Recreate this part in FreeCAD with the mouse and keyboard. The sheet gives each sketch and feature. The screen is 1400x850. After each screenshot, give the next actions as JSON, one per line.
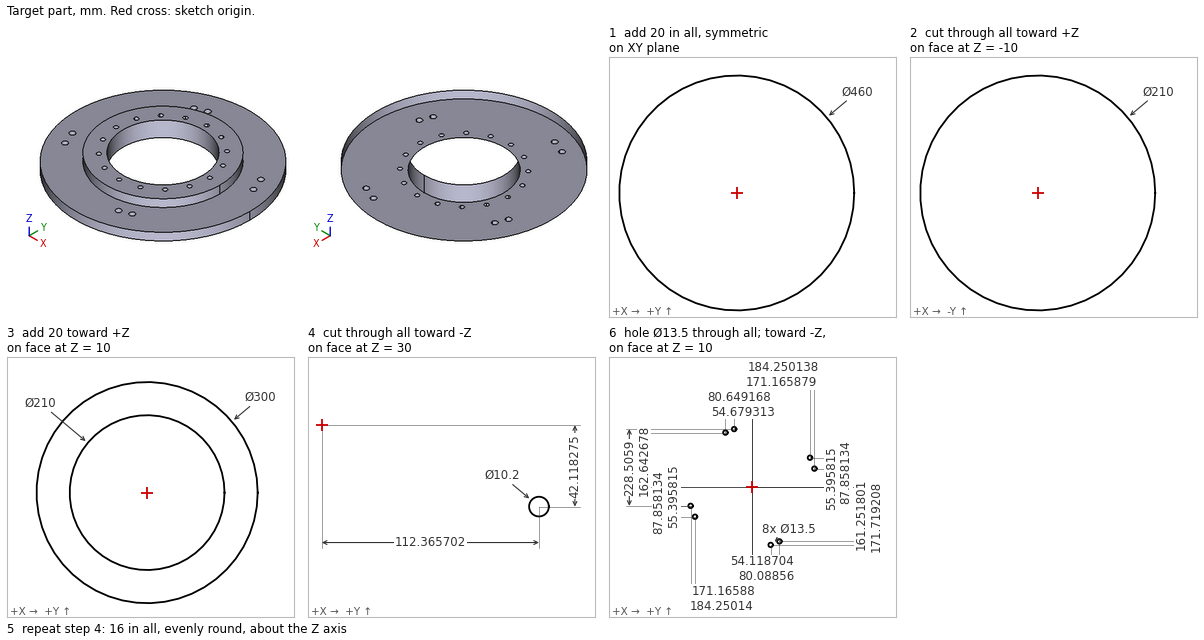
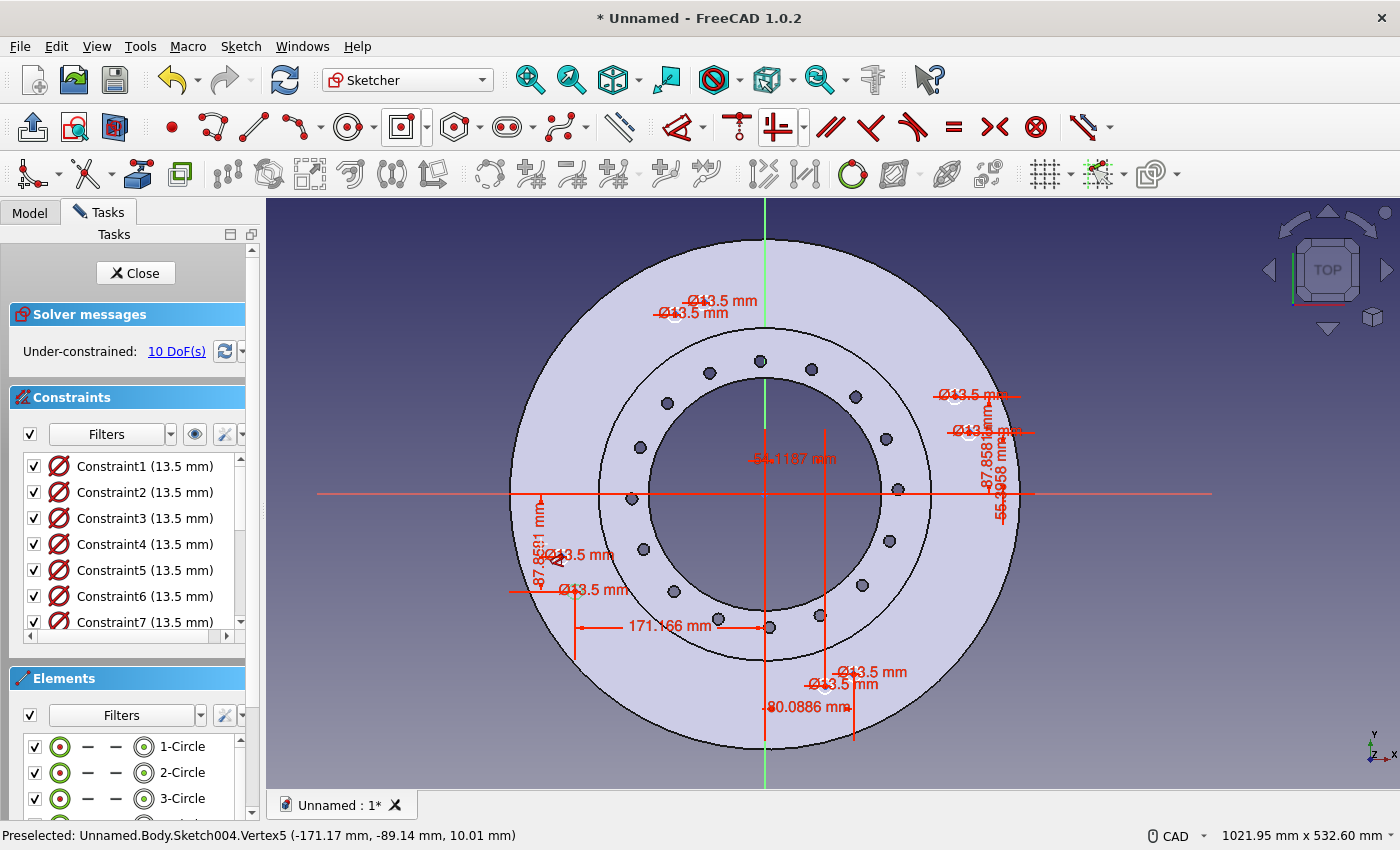
{"action": "left_click", "coordinate": [561, 557]}
{"action": "left_click", "coordinate": [663, 591]}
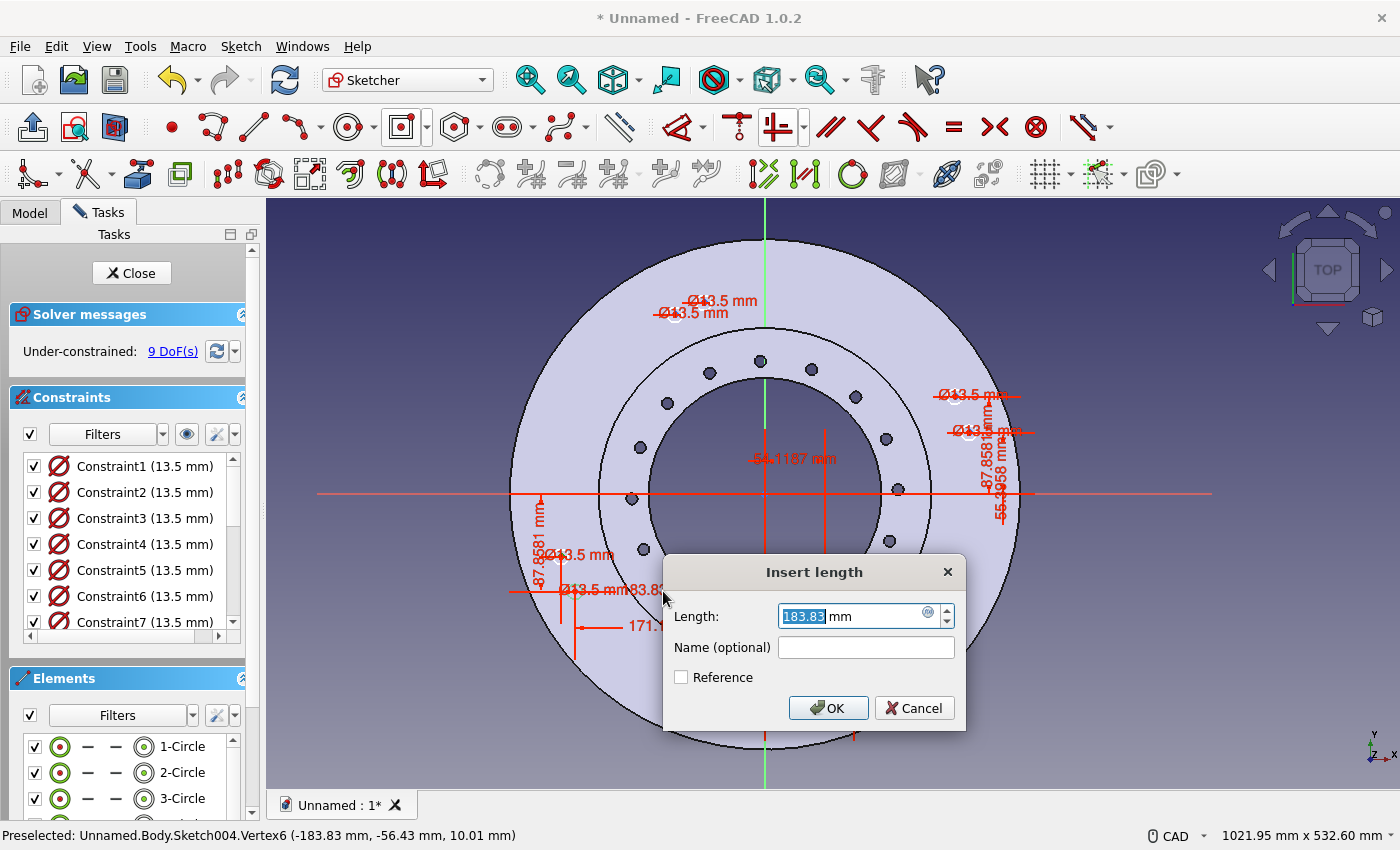
{"action": "type", "text": "184.25014"}
{"action": "key", "text": "Return"}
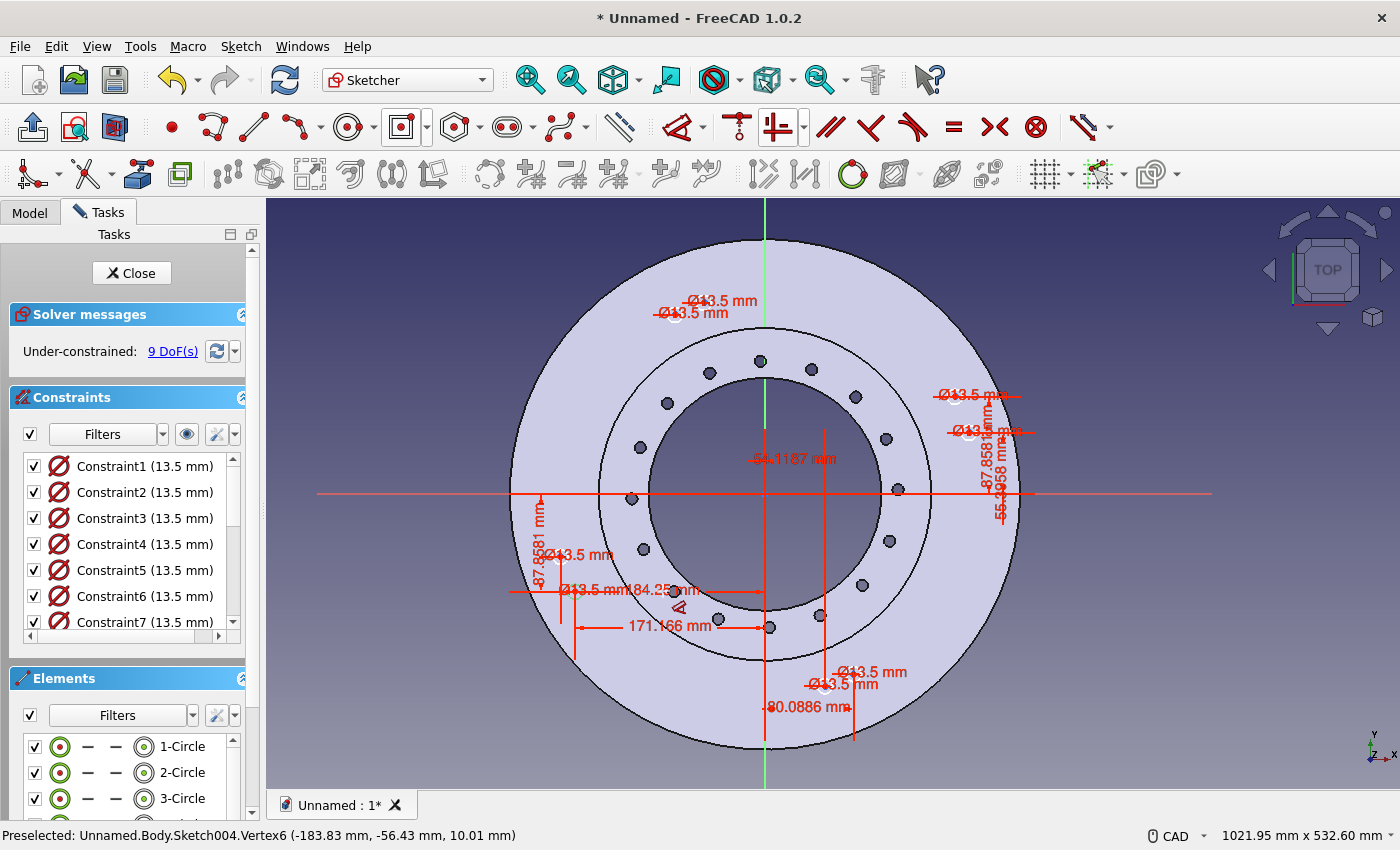
{"action": "left_click", "coordinate": [561, 557]}
{"action": "left_click", "coordinate": [527, 511]}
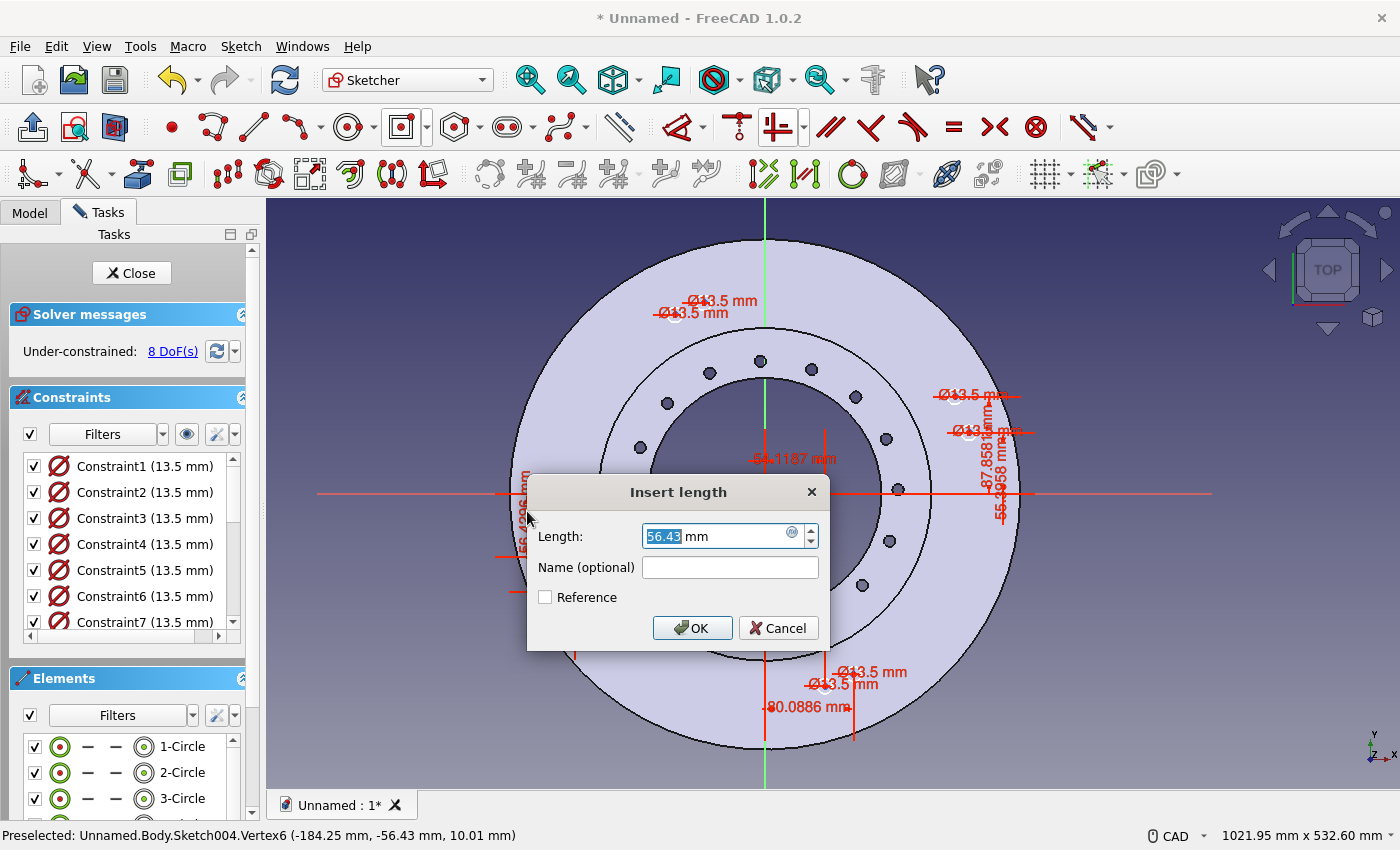
{"action": "type", "text": "55.395815"}
{"action": "key", "text": "Return"}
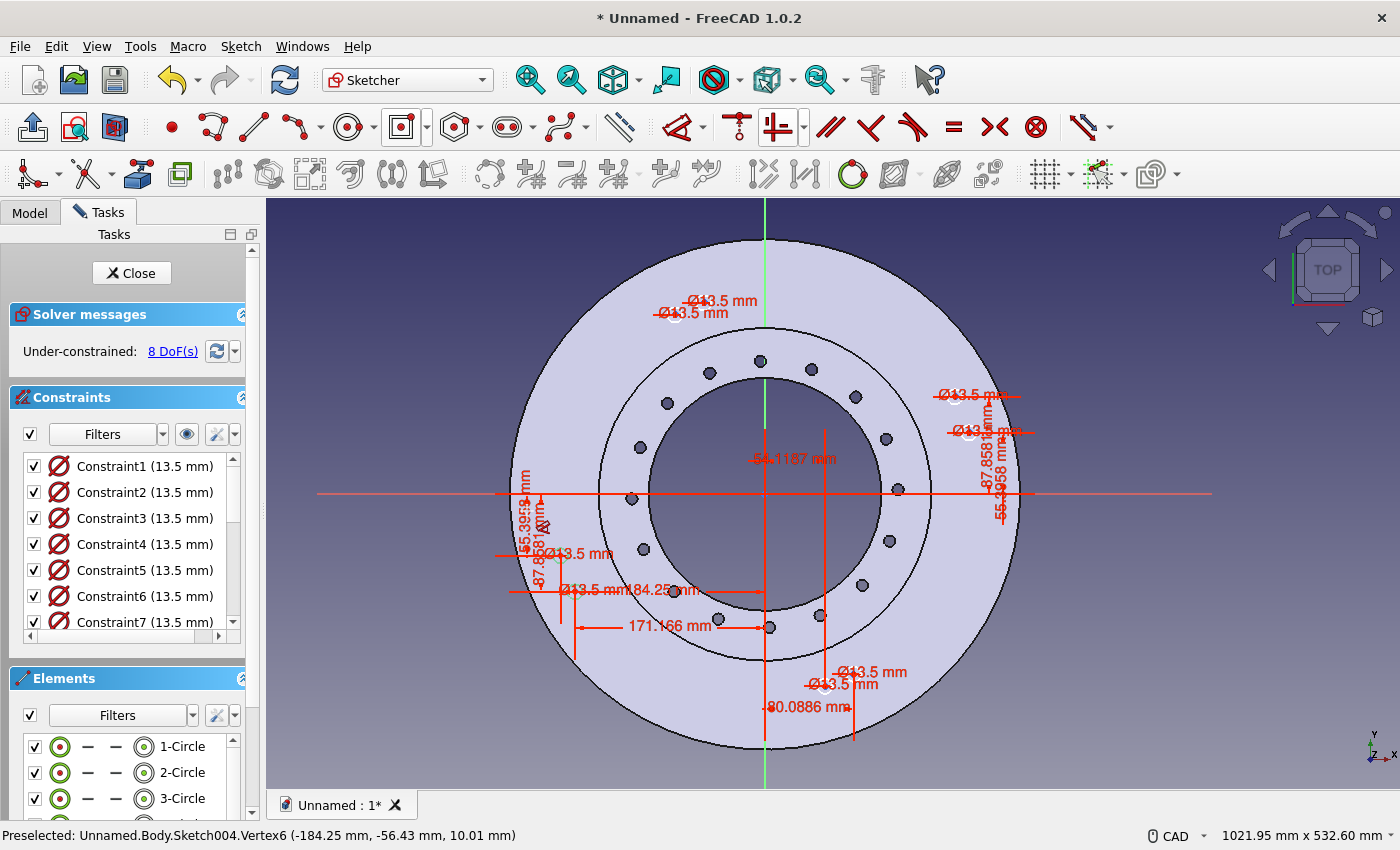
{"action": "left_click", "coordinate": [675, 315]}
{"action": "left_click", "coordinate": [720, 281]}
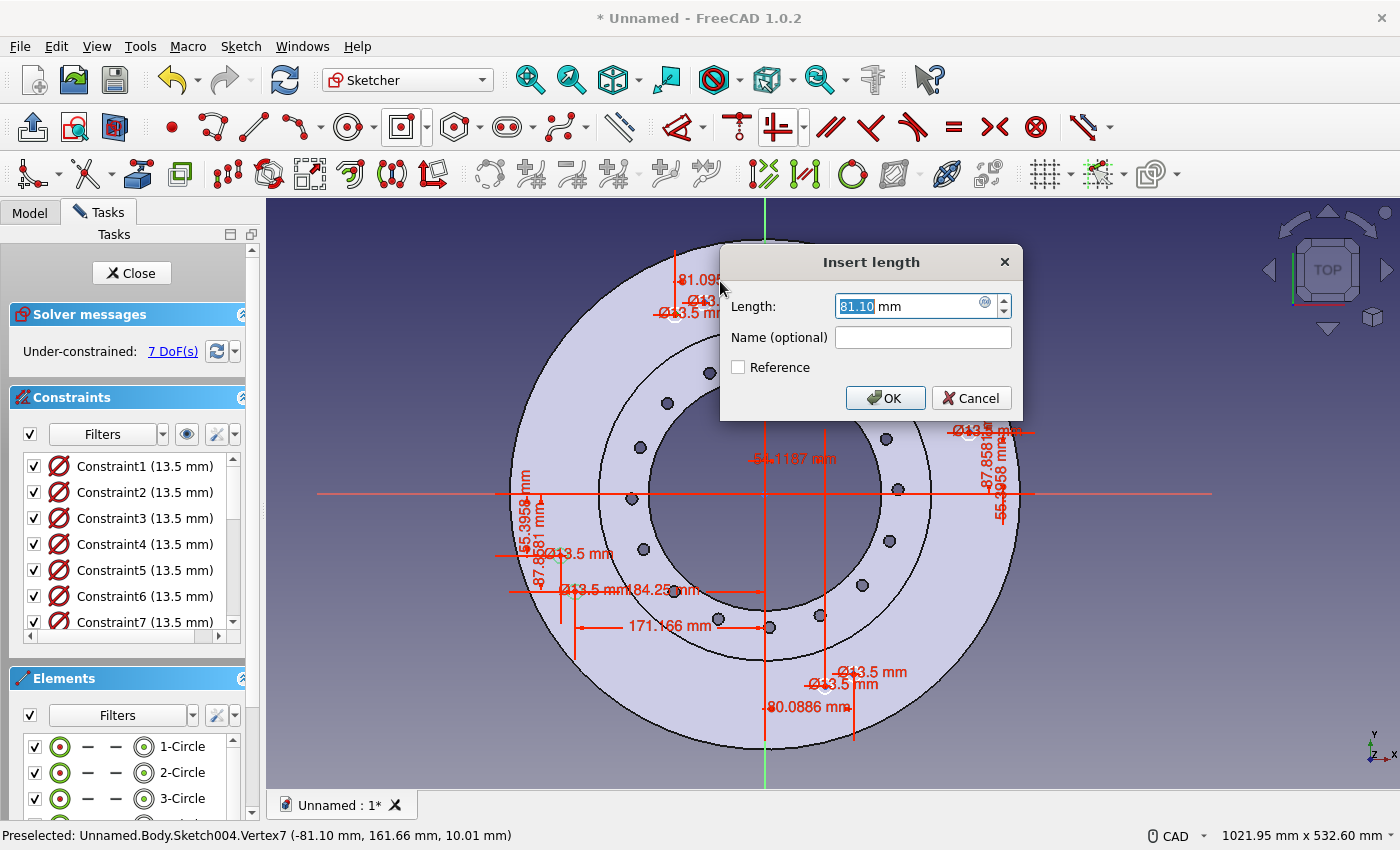
{"action": "type", "text": "80.649168"}
{"action": "key", "text": "Return"}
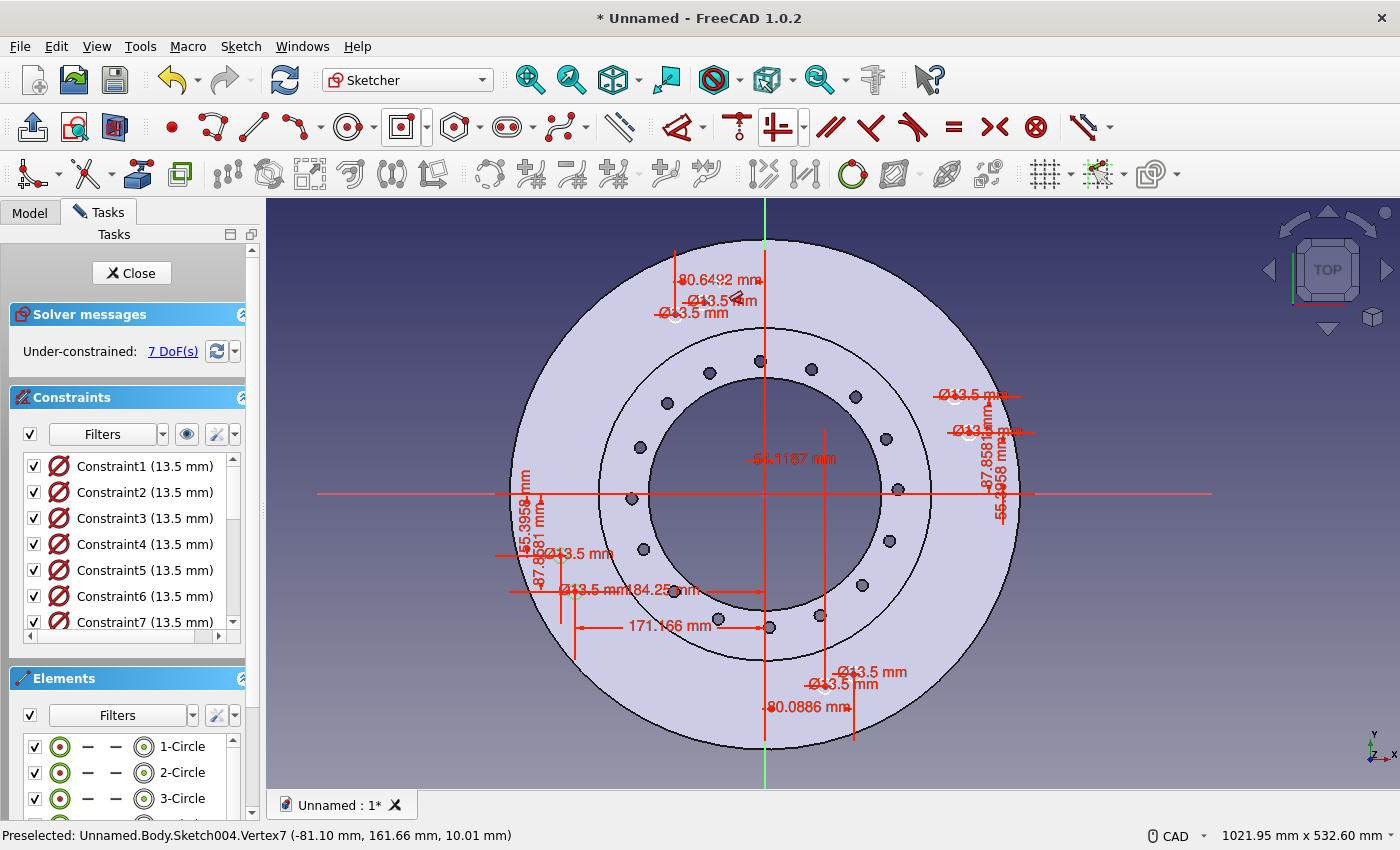
{"action": "left_click", "coordinate": [704, 303]}
{"action": "left_click", "coordinate": [734, 528]}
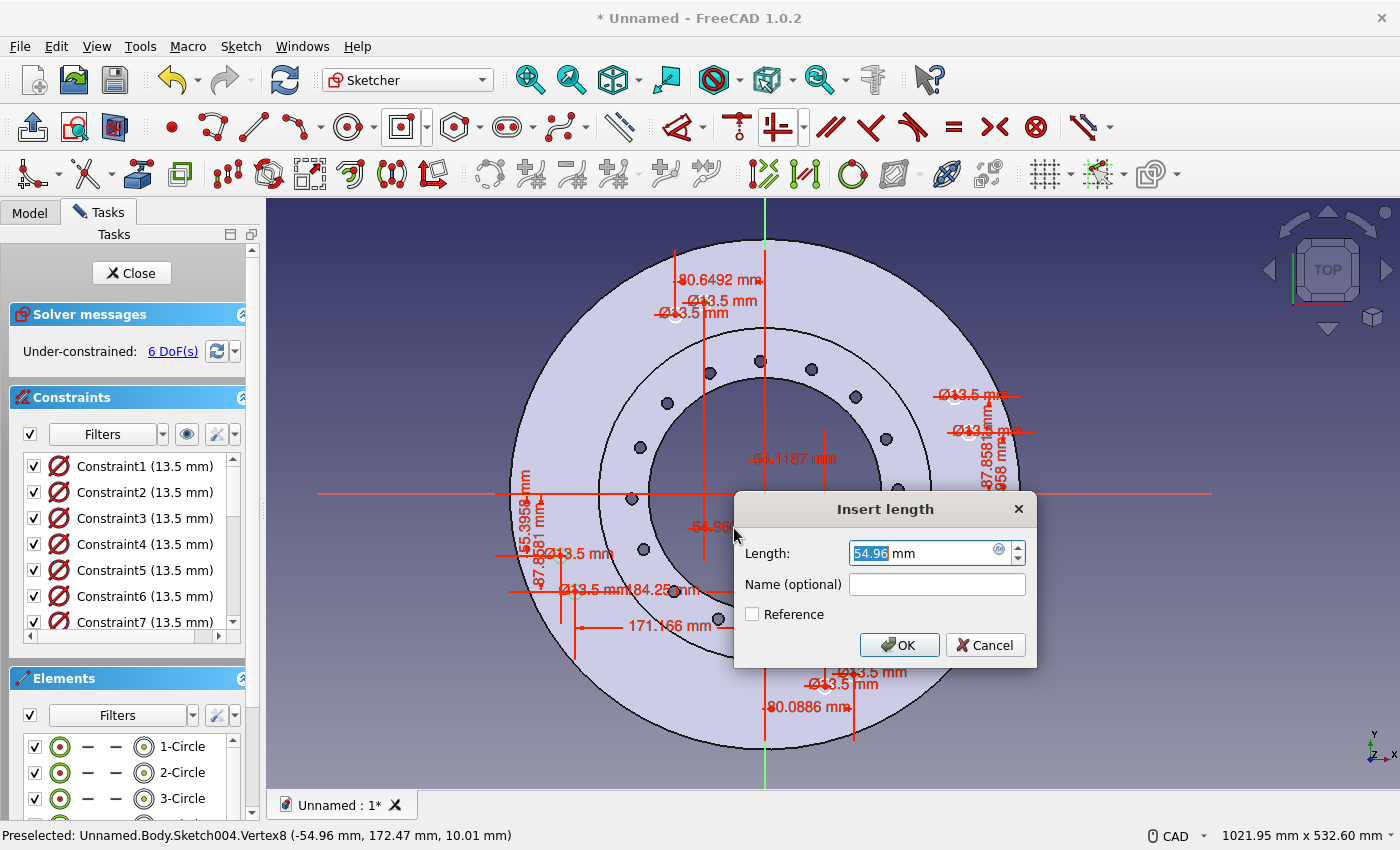
{"action": "type", "text": "54.679313"}
{"action": "key", "text": "Return"}